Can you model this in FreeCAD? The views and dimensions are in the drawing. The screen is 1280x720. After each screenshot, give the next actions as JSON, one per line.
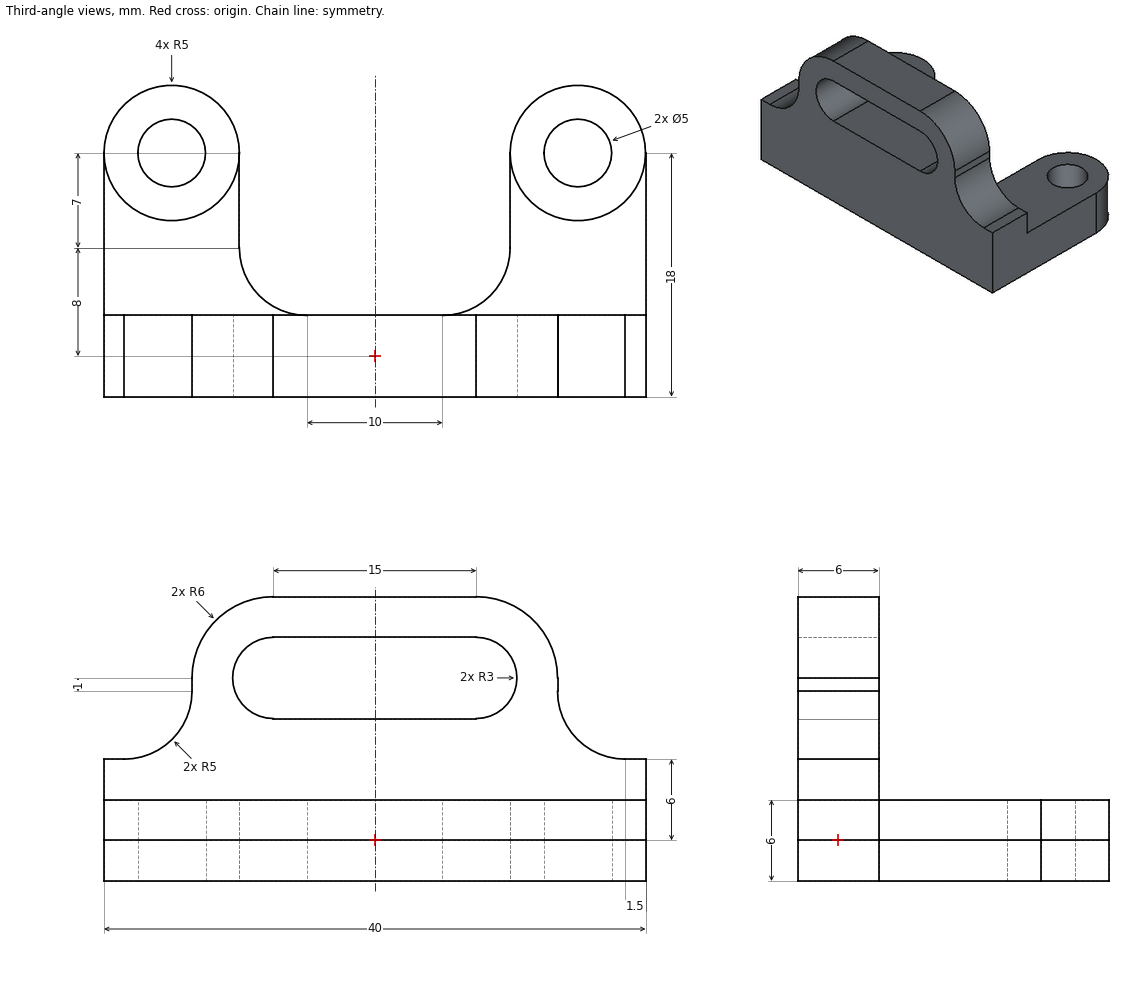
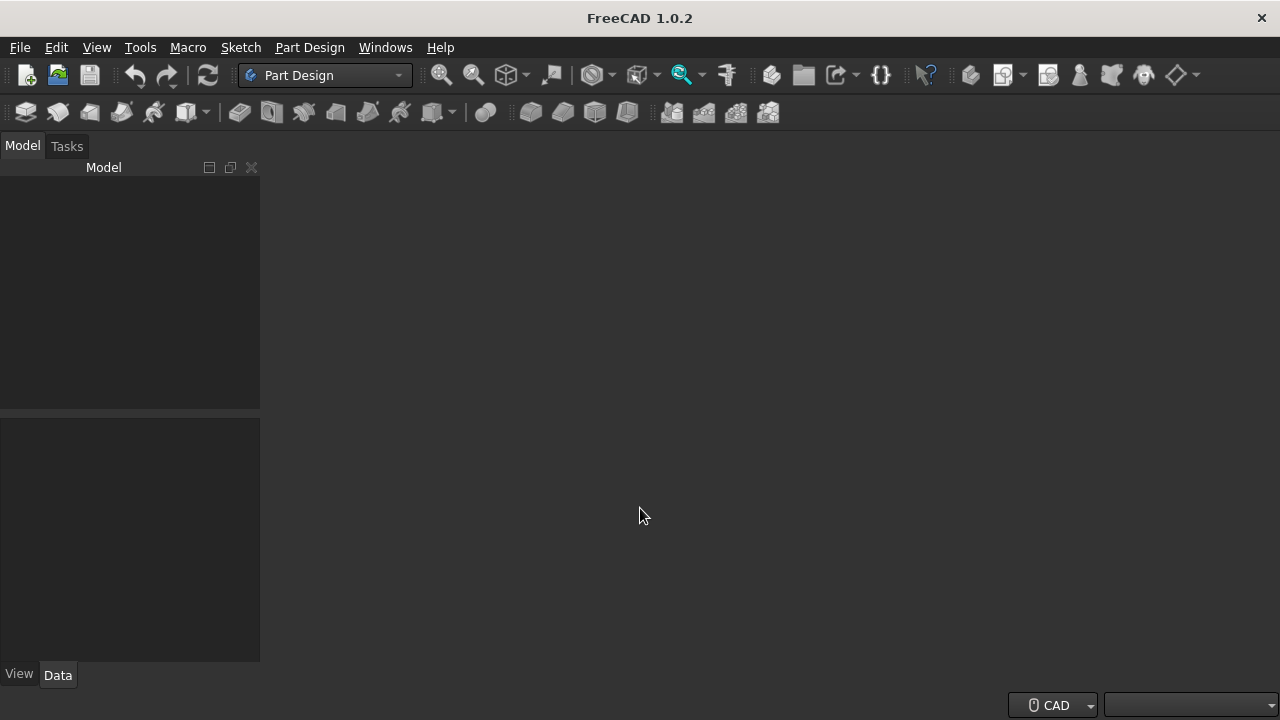
{"action": "left_click", "coordinate": [26, 76]}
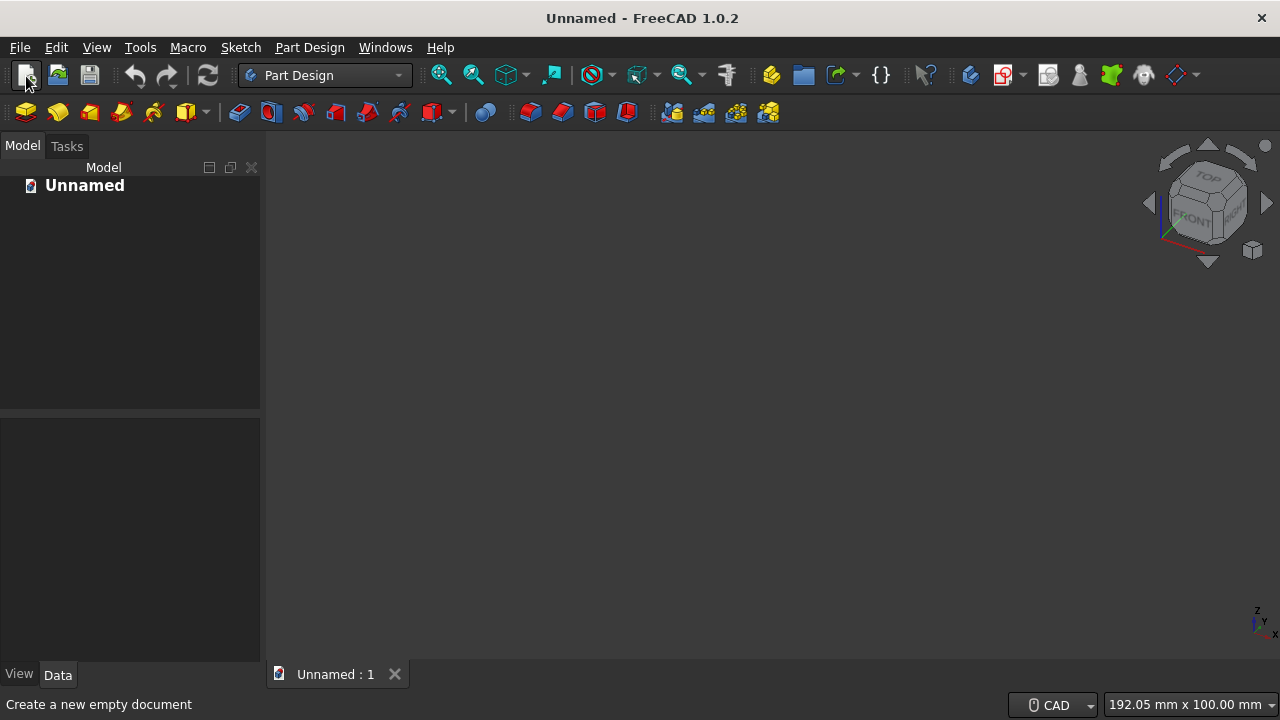
{"action": "left_click", "coordinate": [1004, 76]}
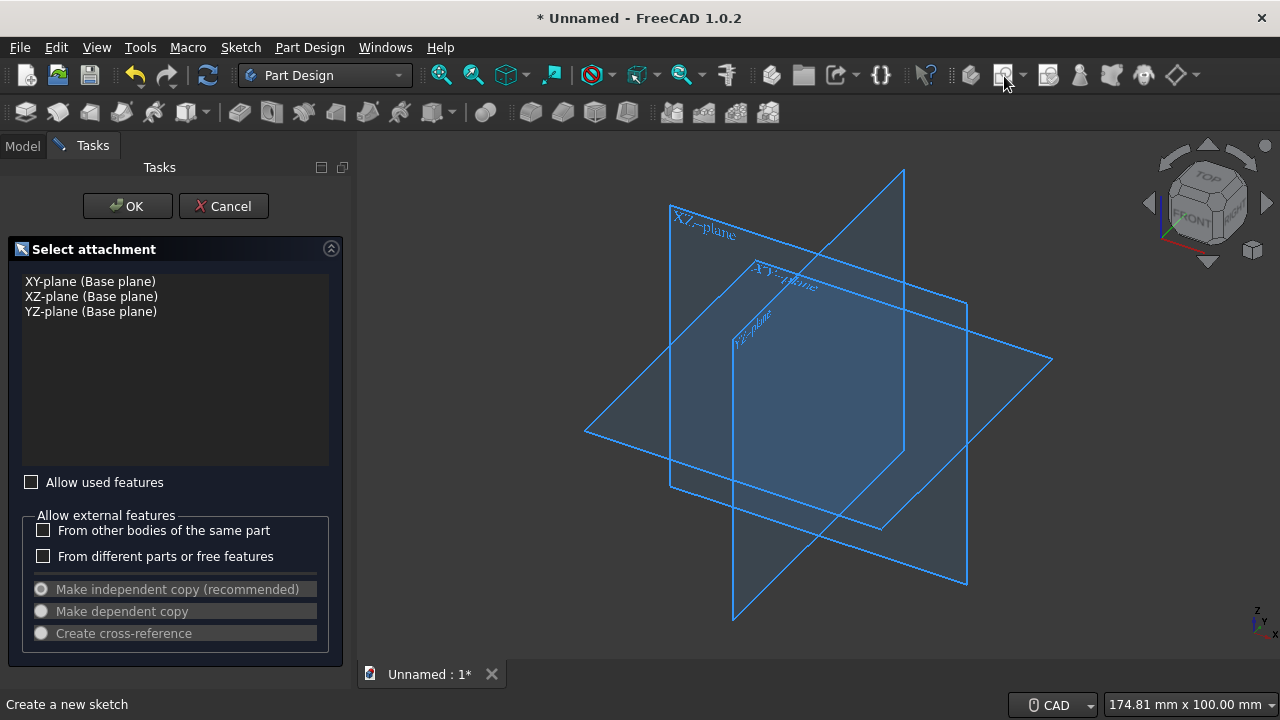
{"action": "left_click", "coordinate": [82, 296]}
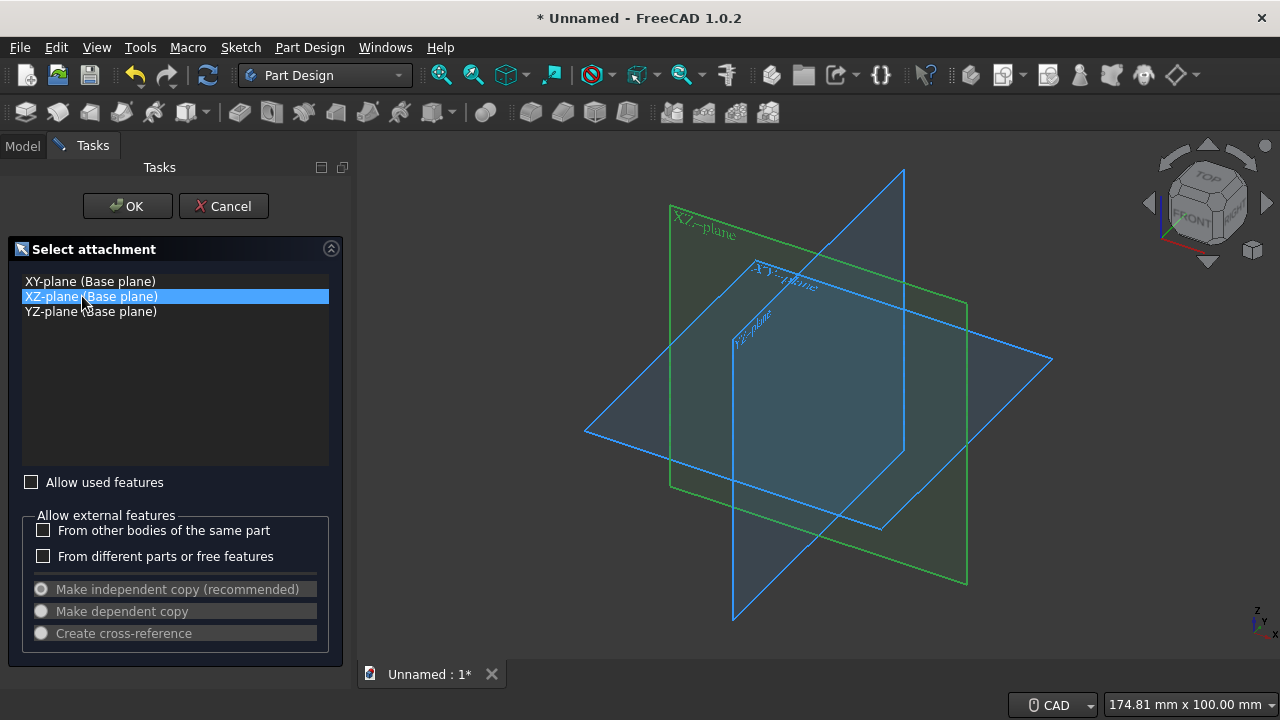
{"action": "left_click", "coordinate": [128, 206]}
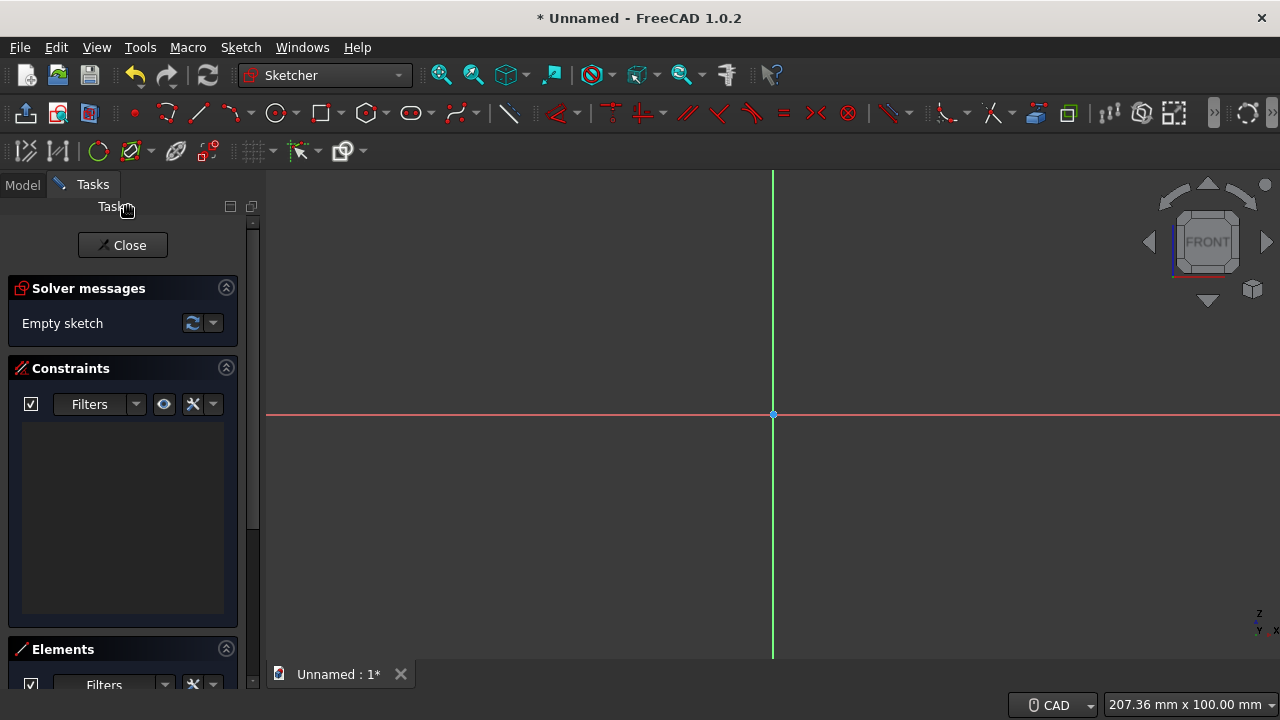
{"action": "scroll", "coordinate": [813, 345], "scroll_direction": "up", "scroll_amount": 5}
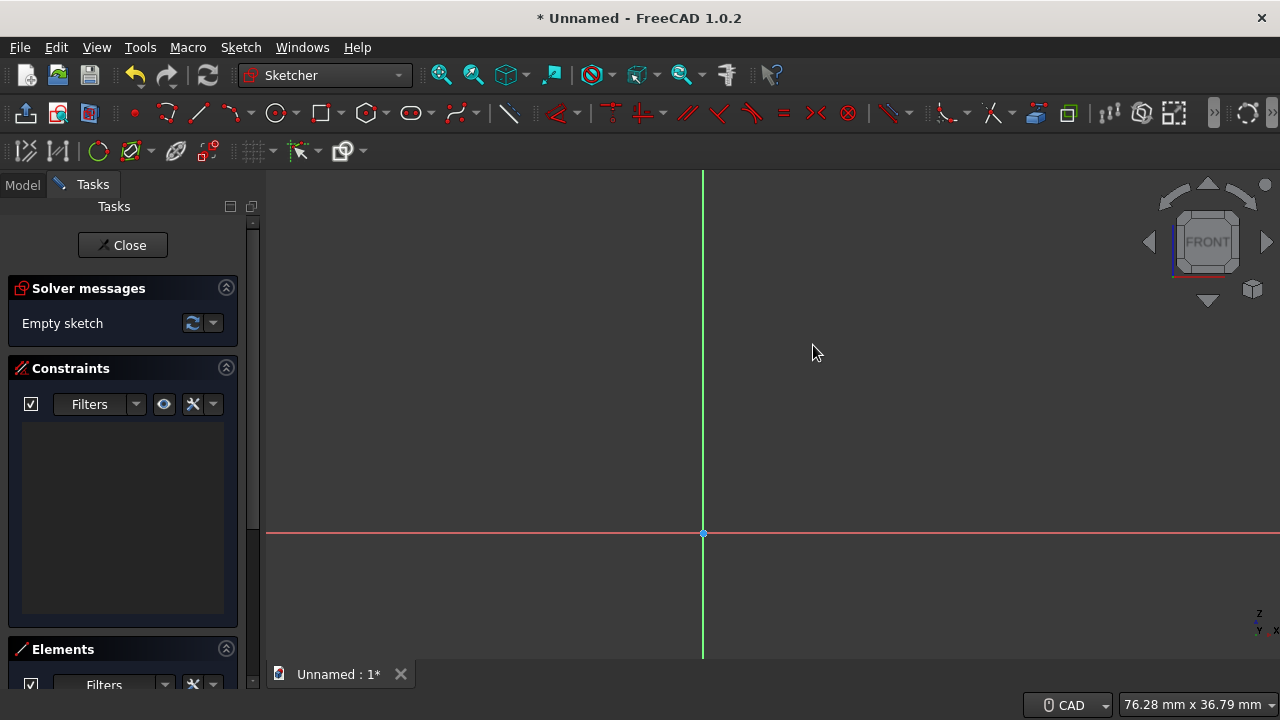
{"action": "key", "text": "g l"}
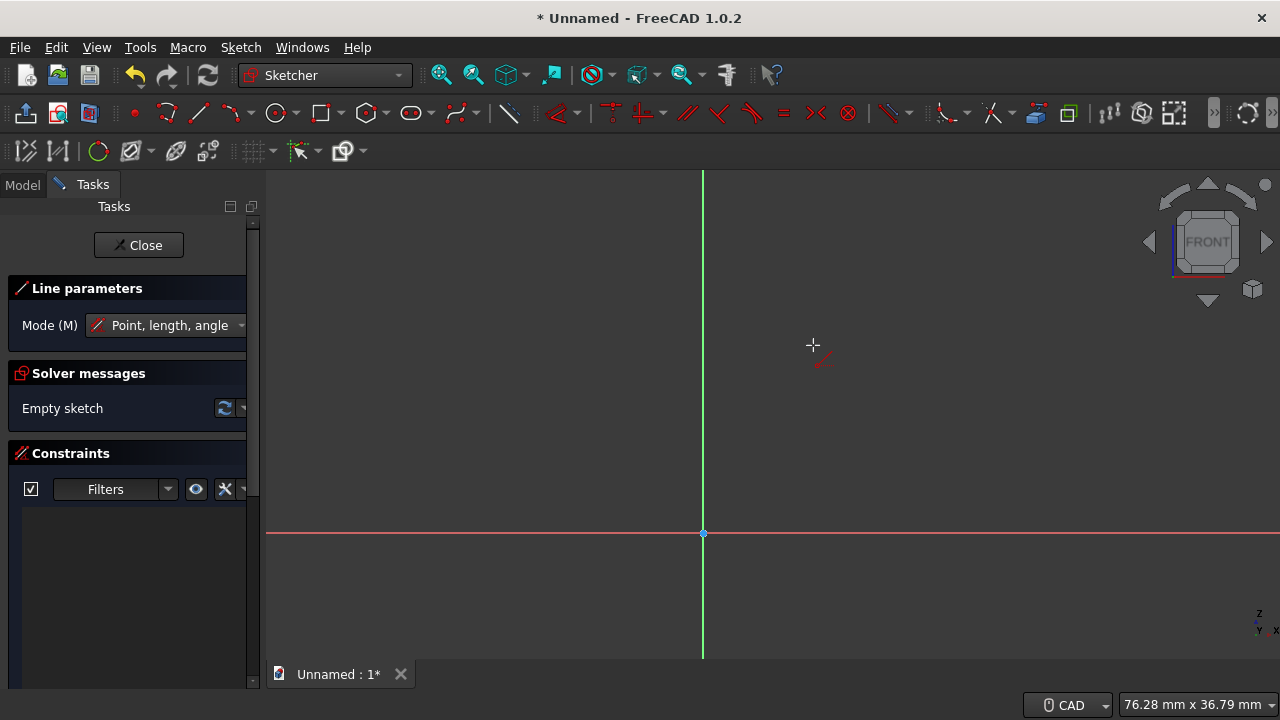
{"action": "left_click", "coordinate": [524, 387]}
{"action": "left_click", "coordinate": [524, 374]}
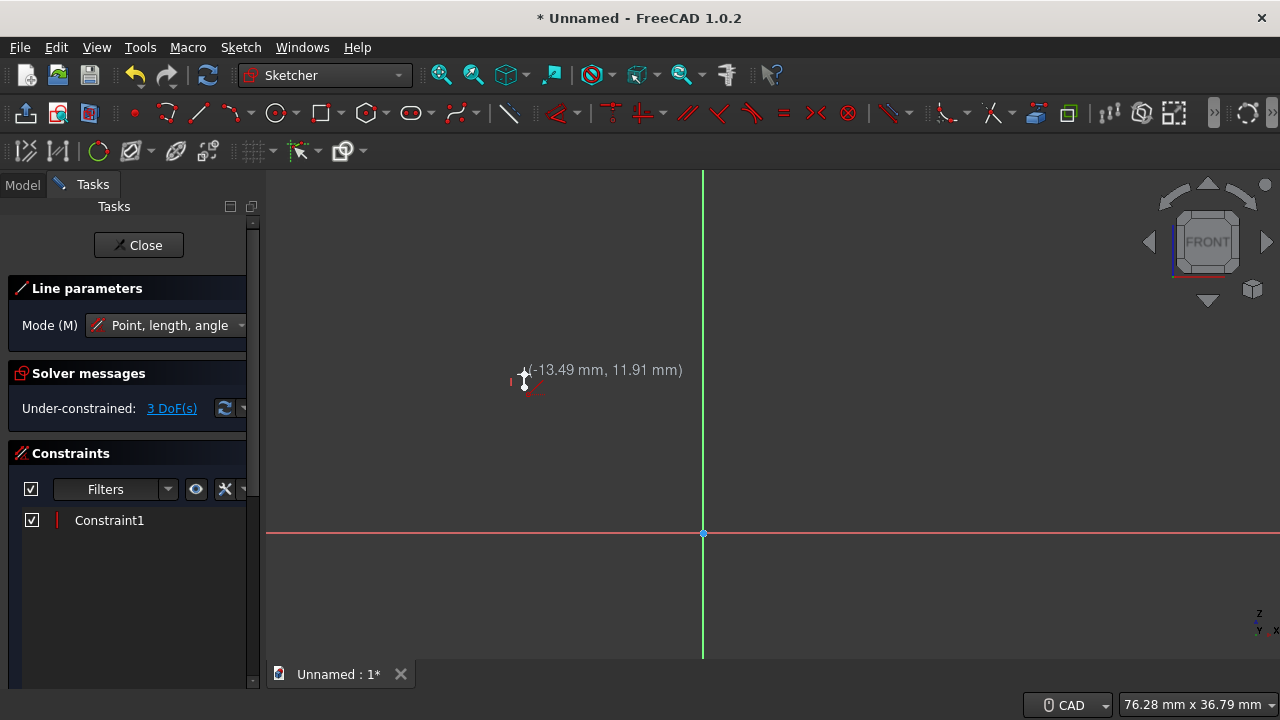
{"action": "left_click", "coordinate": [604, 294]}
{"action": "left_click", "coordinate": [803, 294]}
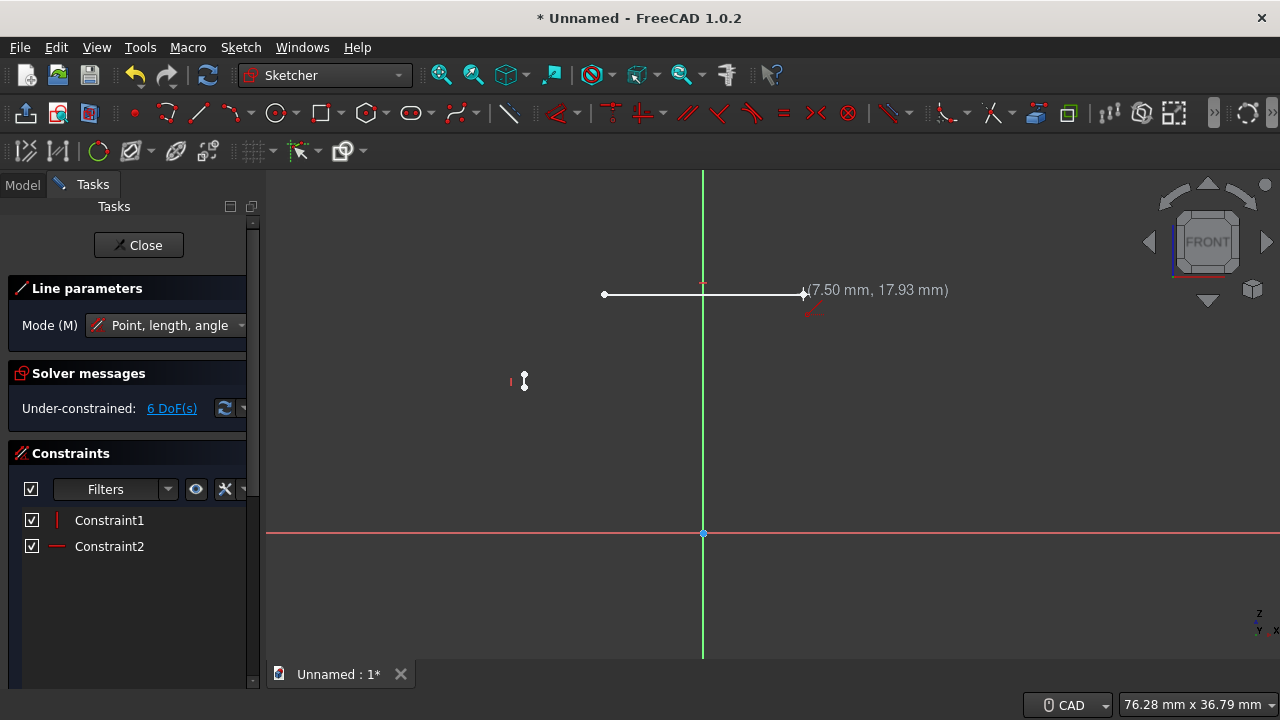
{"action": "left_click", "coordinate": [883, 374]}
{"action": "left_click", "coordinate": [883, 387]}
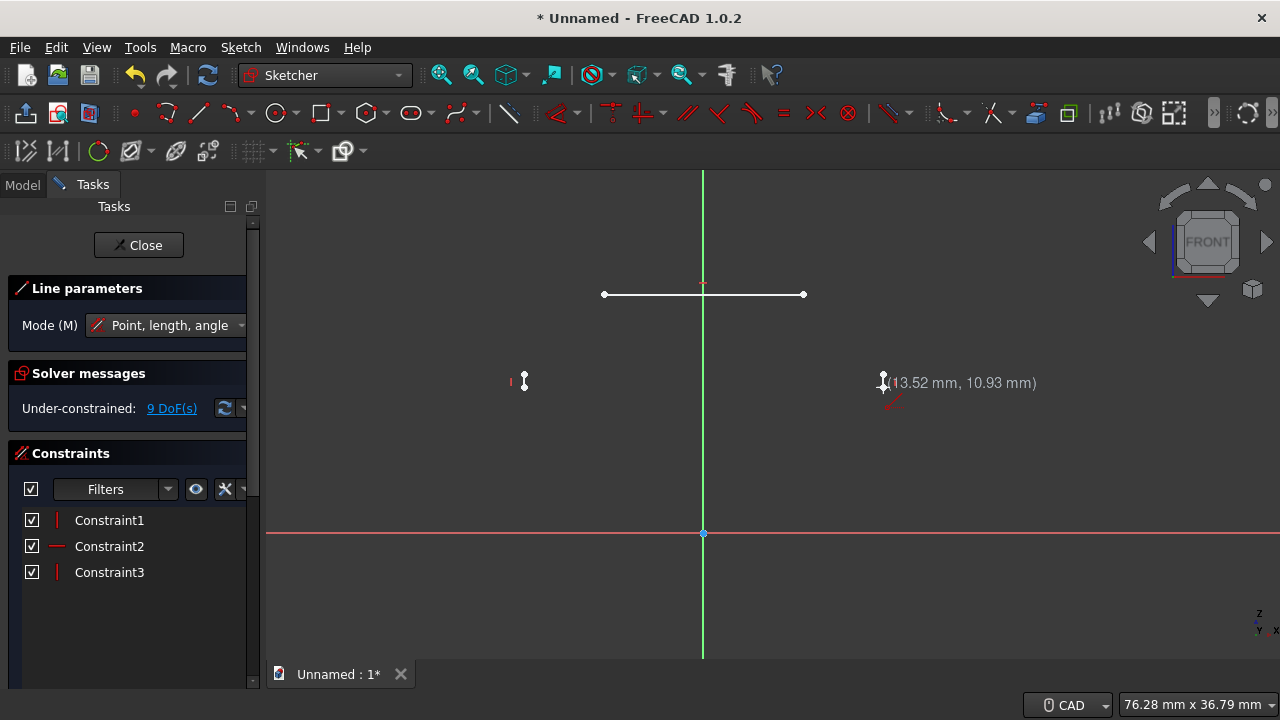
{"action": "left_click", "coordinate": [168, 114]}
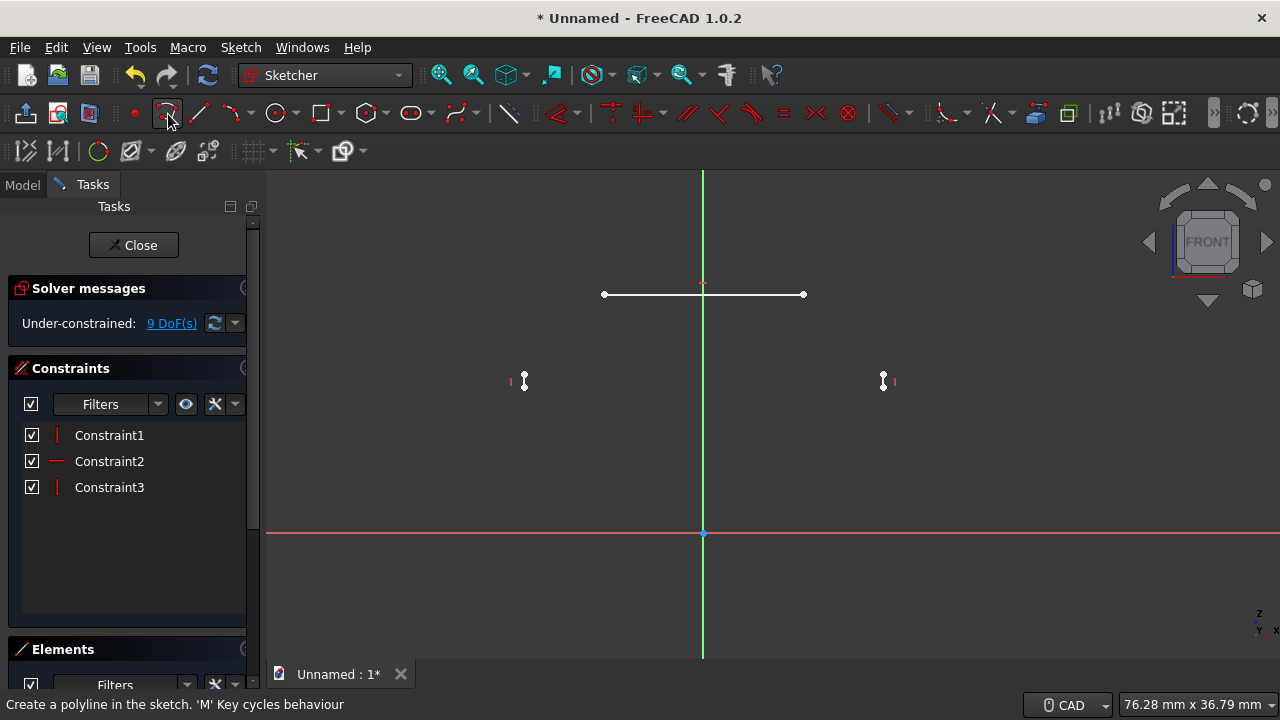
{"action": "left_click", "coordinate": [949, 454]}
{"action": "left_click", "coordinate": [969, 454]}
{"action": "left_click", "coordinate": [969, 533]}
{"action": "left_click", "coordinate": [437, 524]}
{"action": "left_click", "coordinate": [437, 454]}
{"action": "left_click", "coordinate": [457, 454]}
{"action": "right_click", "coordinate": [457, 454]}